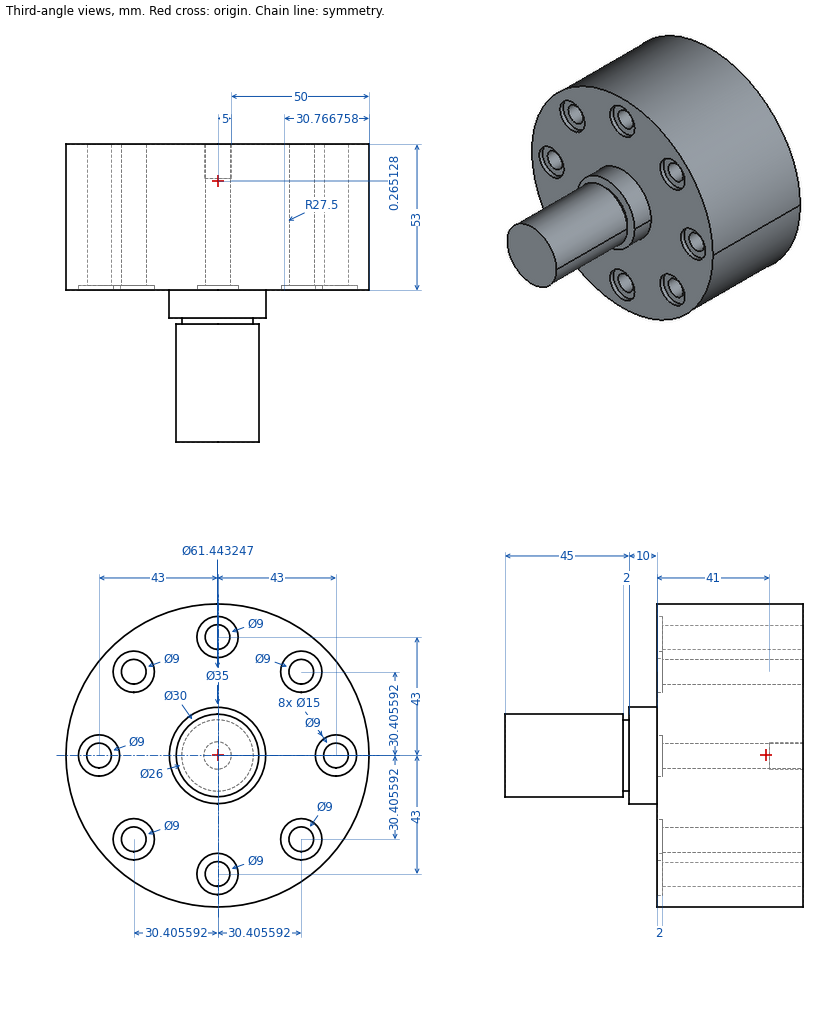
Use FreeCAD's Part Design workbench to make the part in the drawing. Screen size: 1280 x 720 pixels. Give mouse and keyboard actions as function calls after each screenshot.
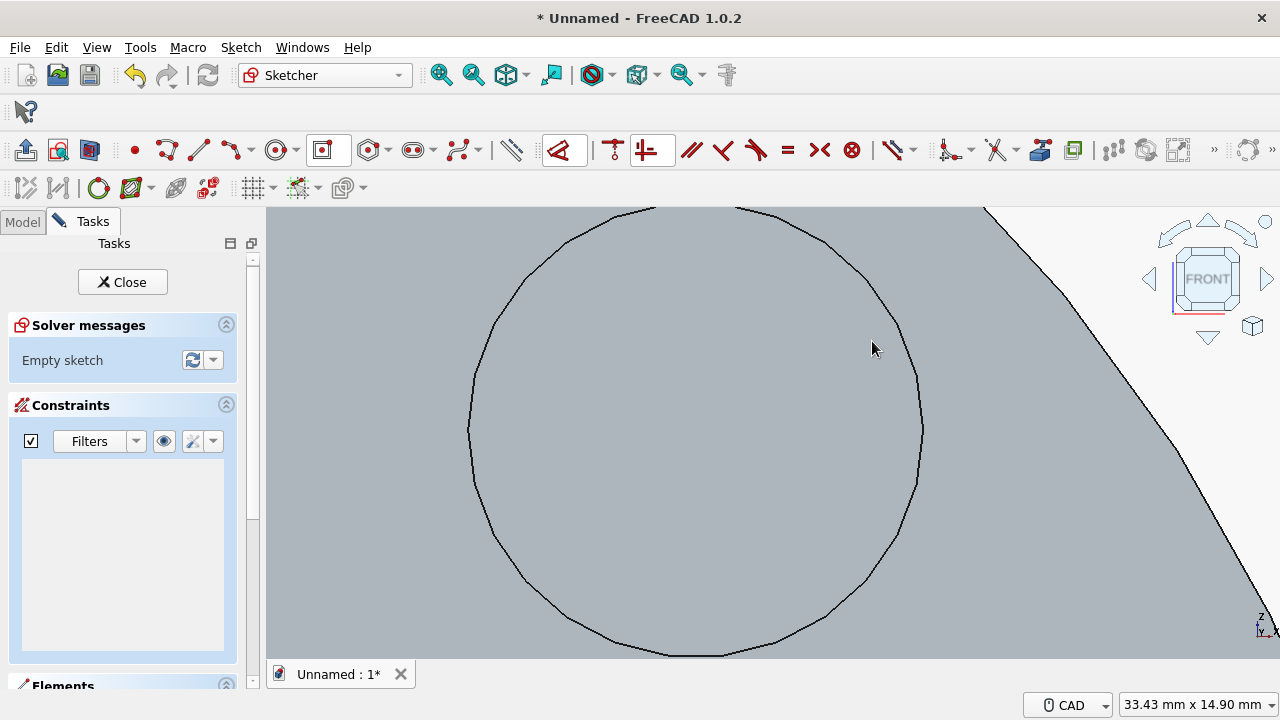
click(276, 150)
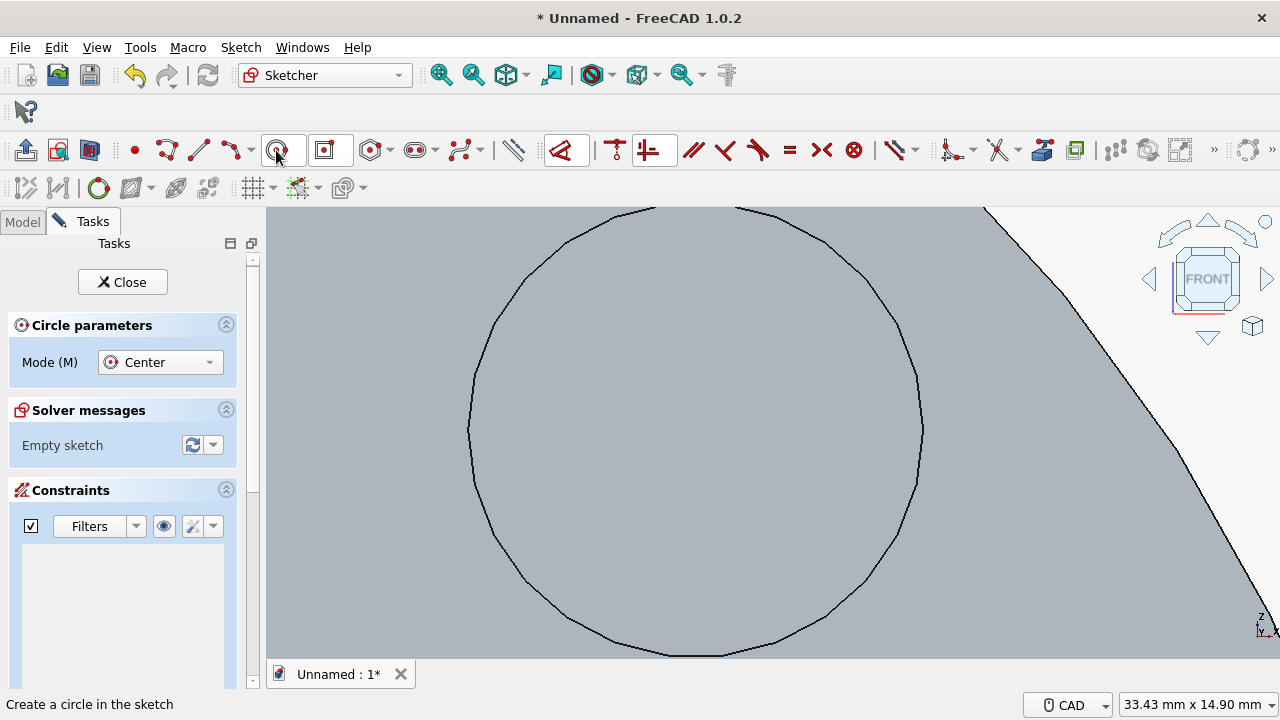
click(696, 430)
move(792, 333)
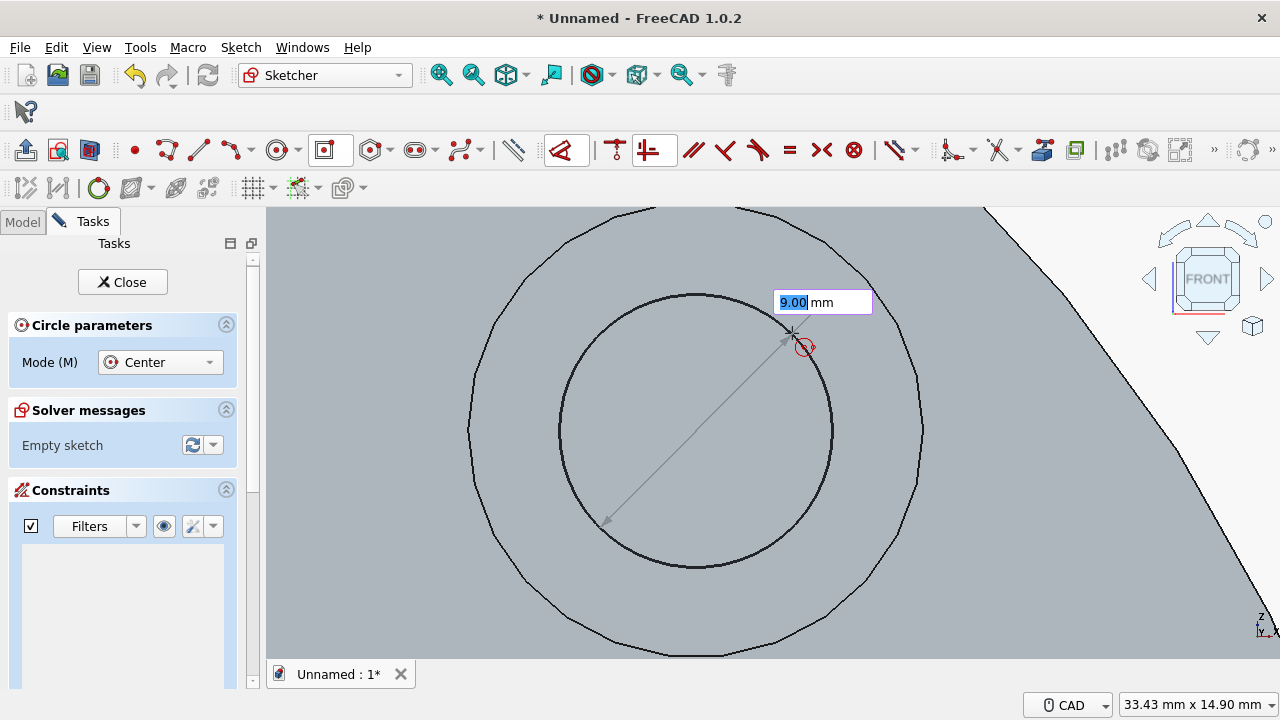
text(9)
key(Return)
key(Escape)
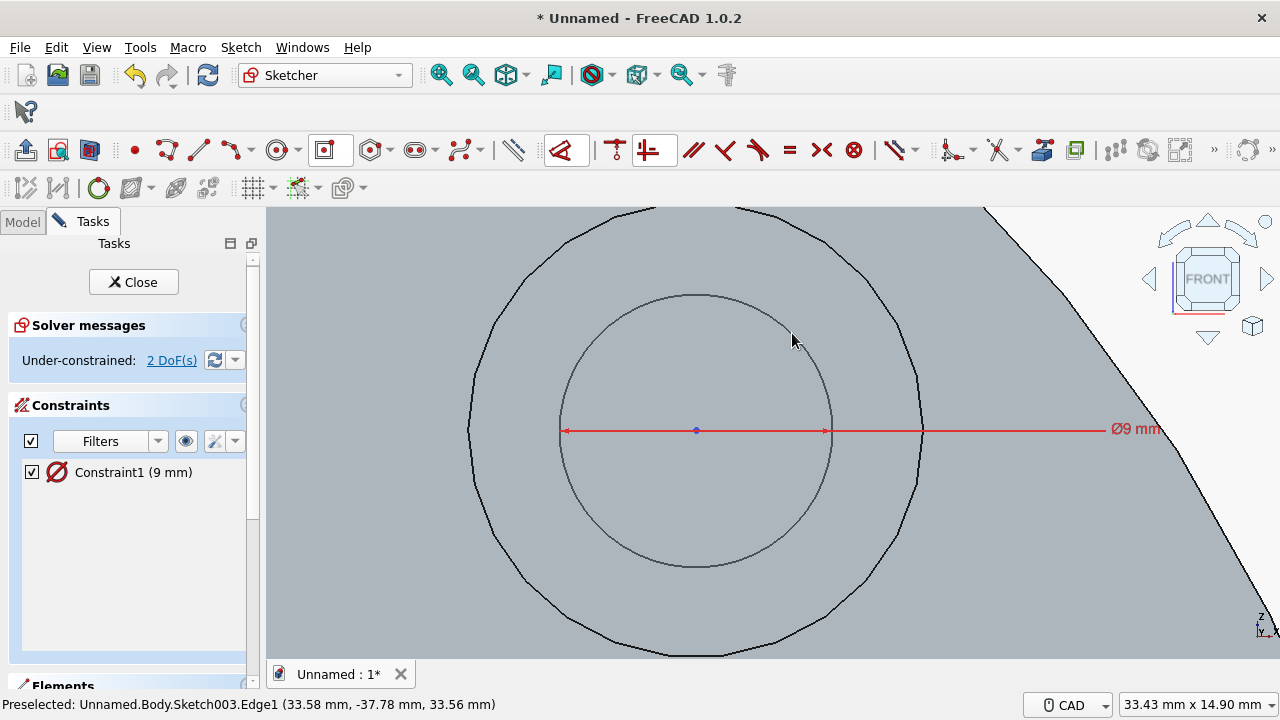
click(696, 431)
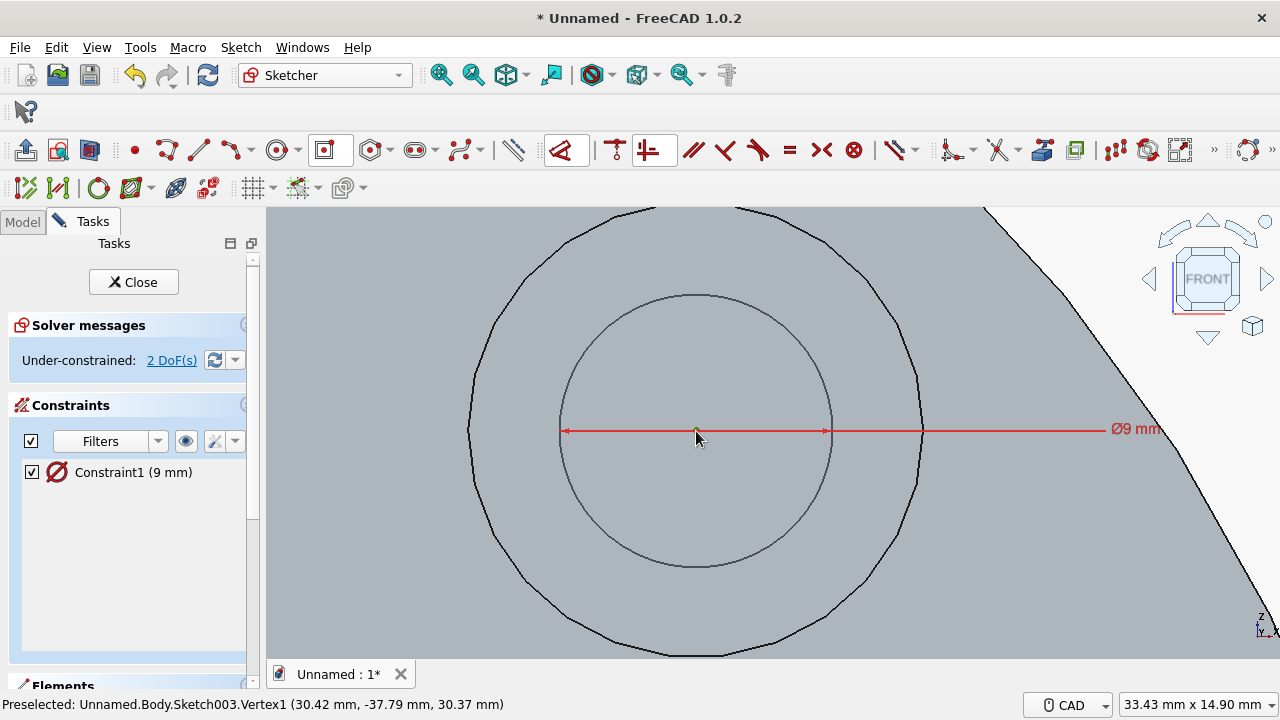
click(584, 150)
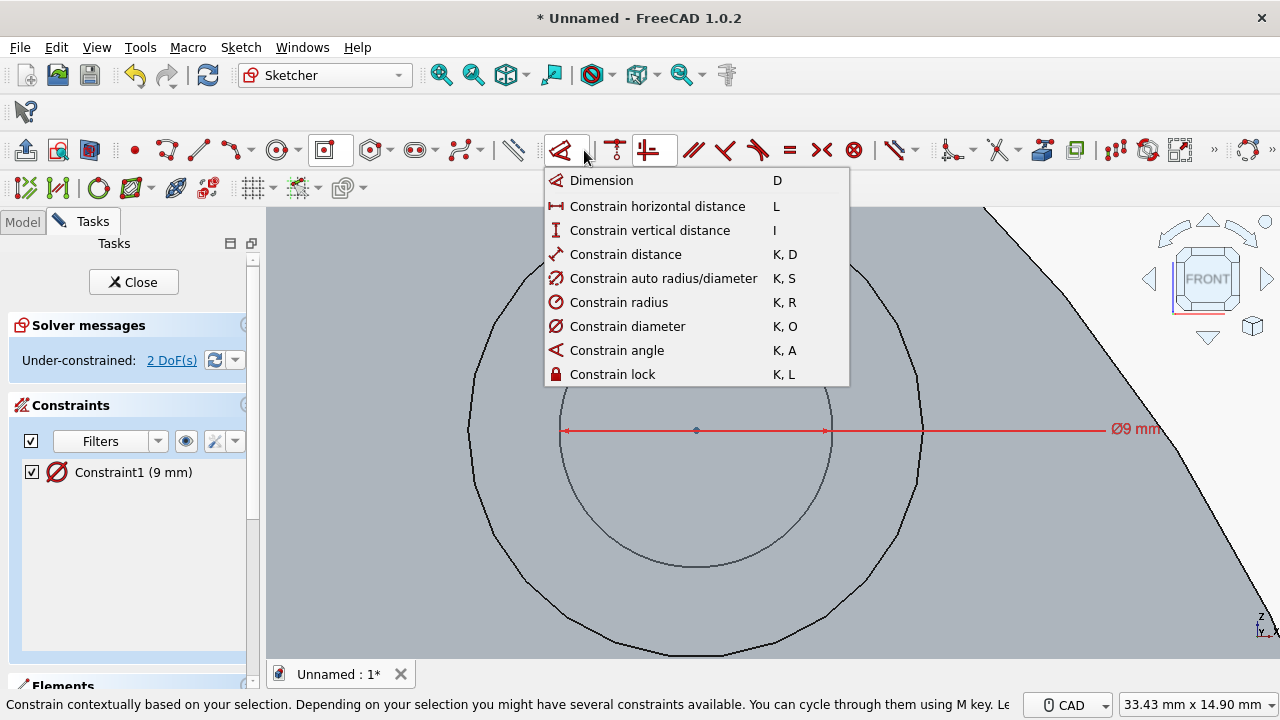
click(697, 206)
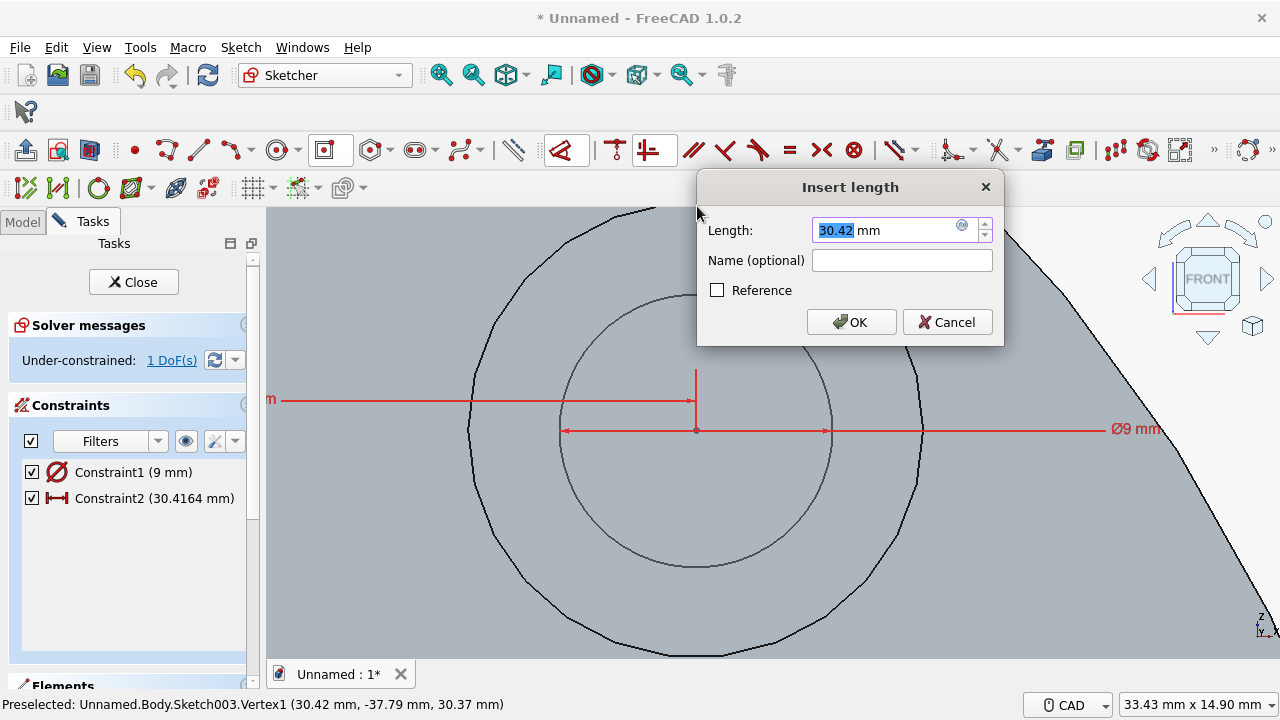
text(30.405592)
key(Return)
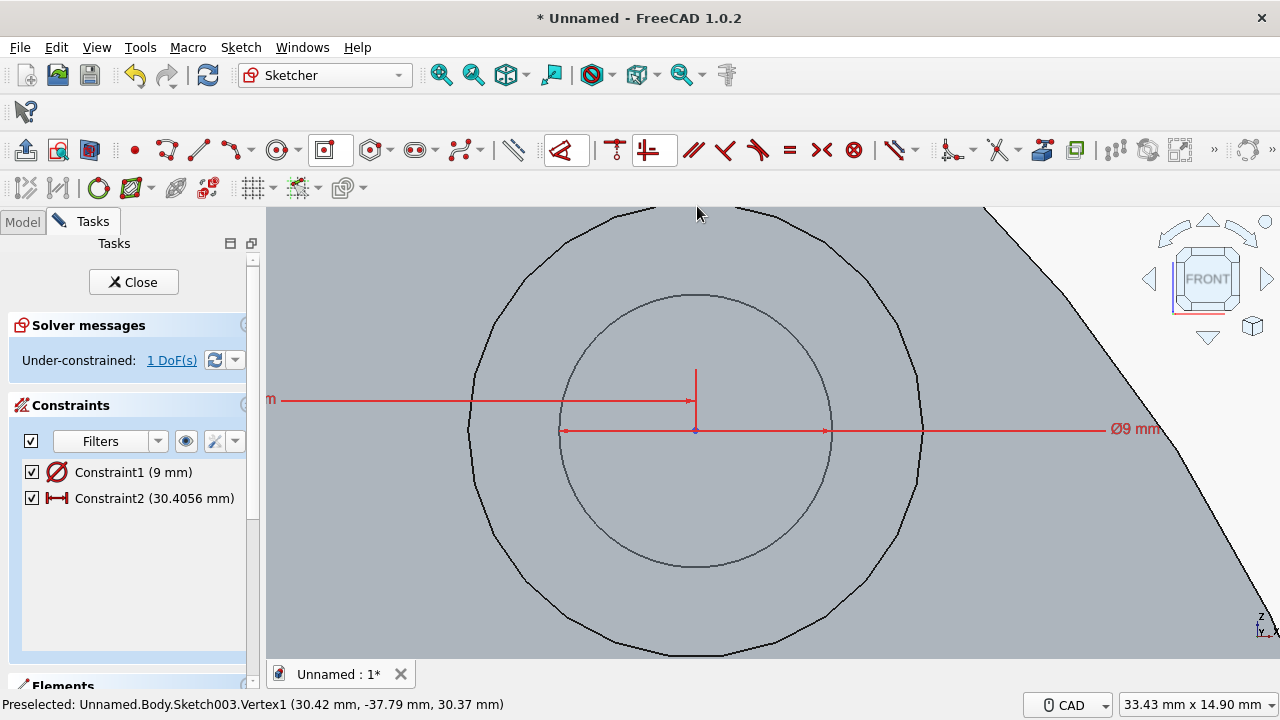
click(696, 431)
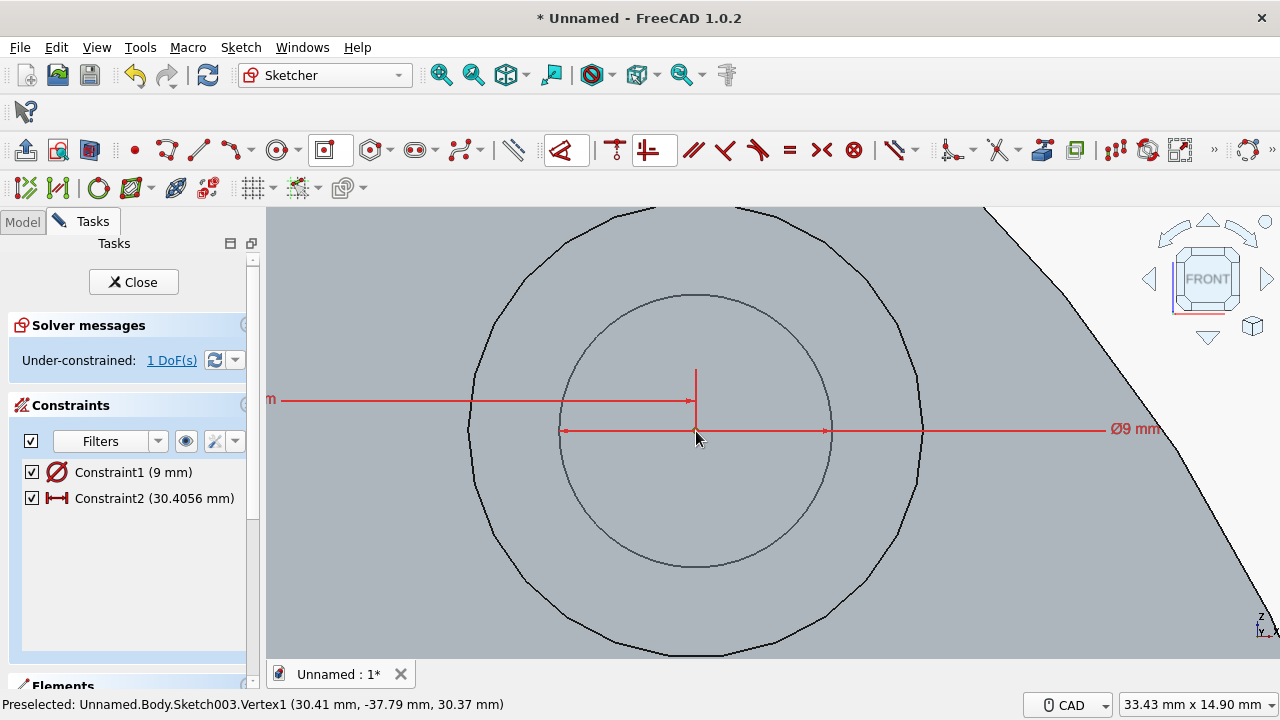
key(i)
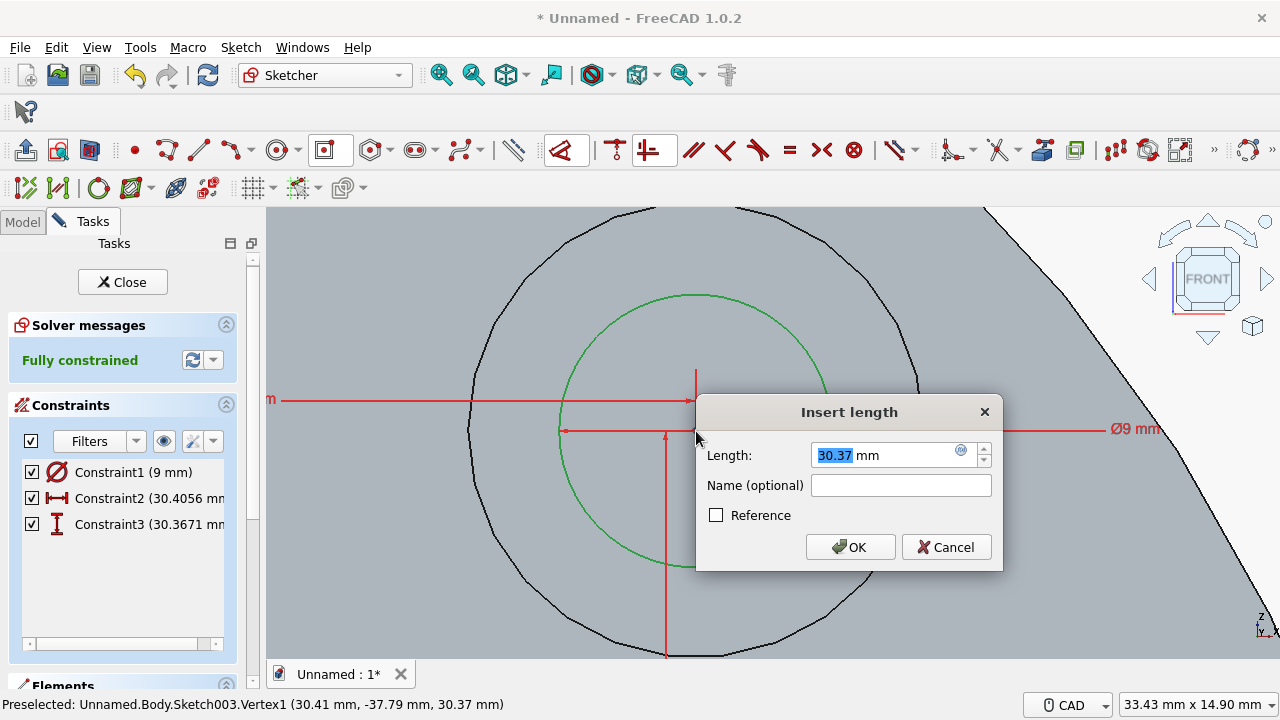
text(30.405592)
key(Return)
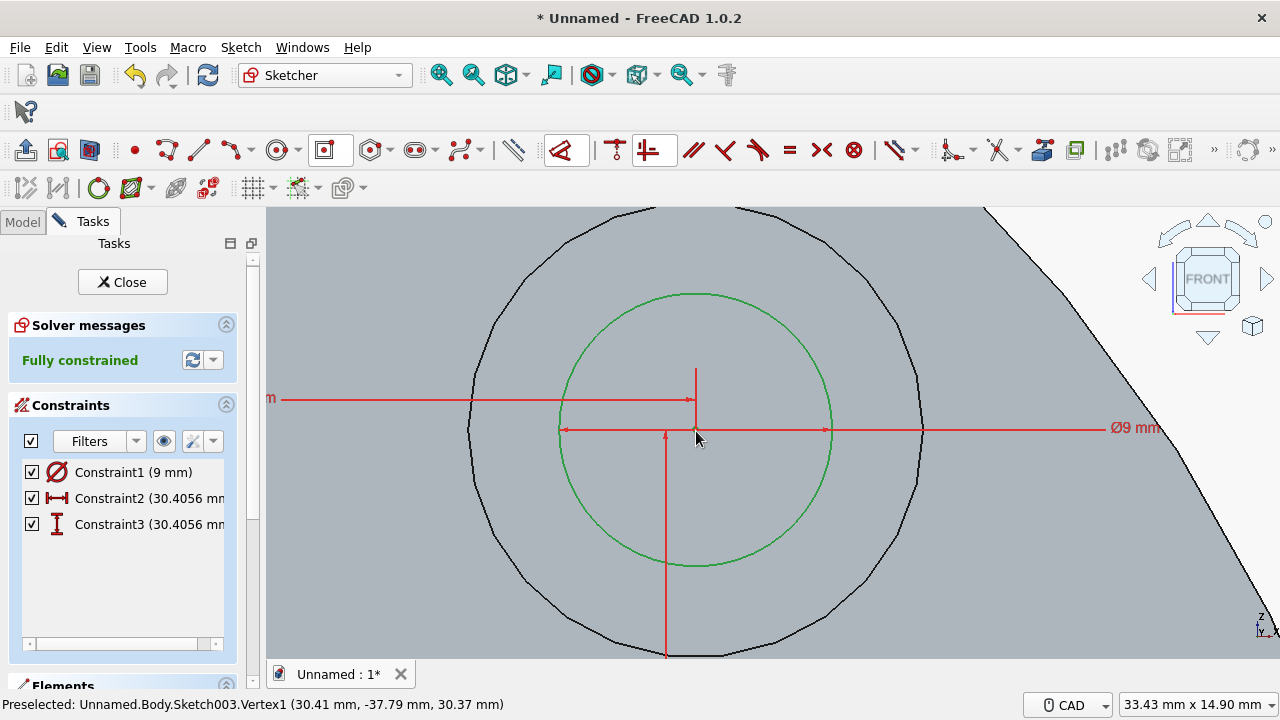
click(123, 282)